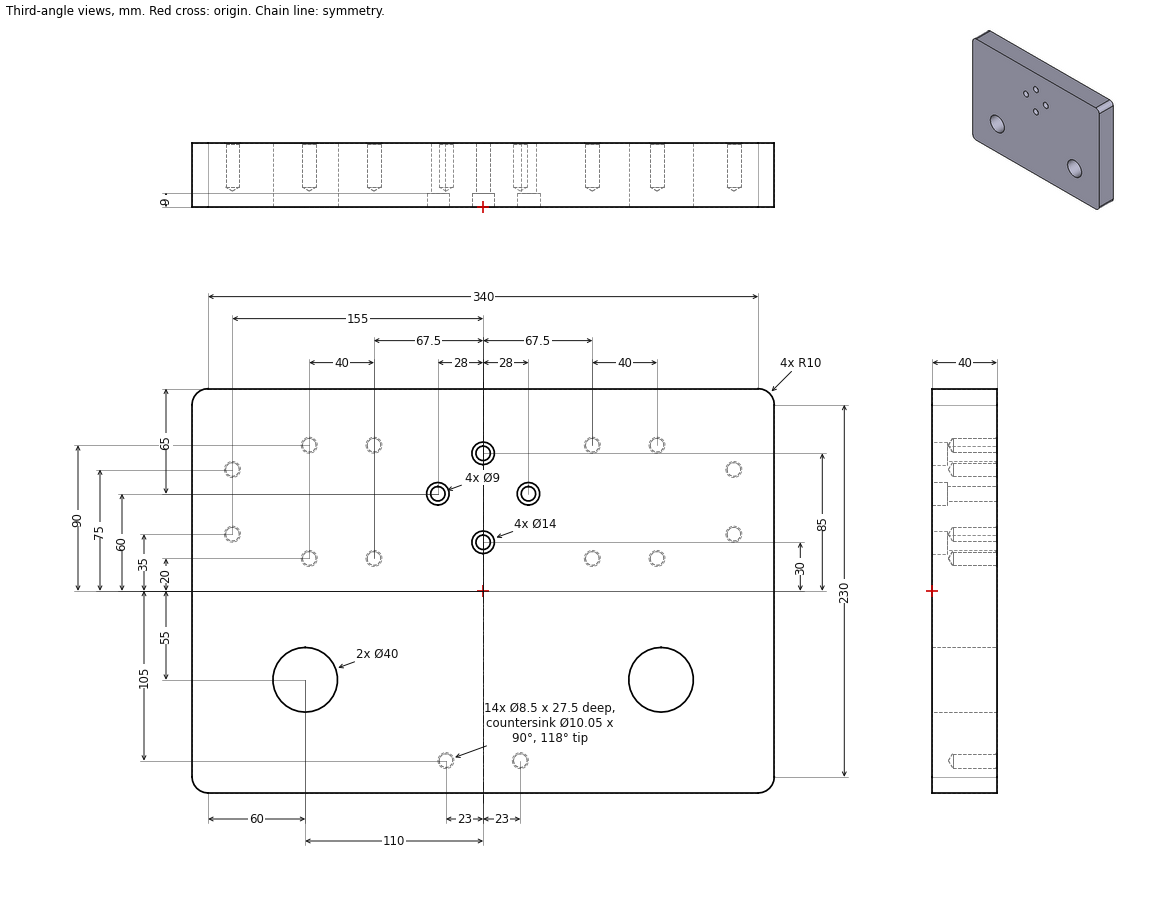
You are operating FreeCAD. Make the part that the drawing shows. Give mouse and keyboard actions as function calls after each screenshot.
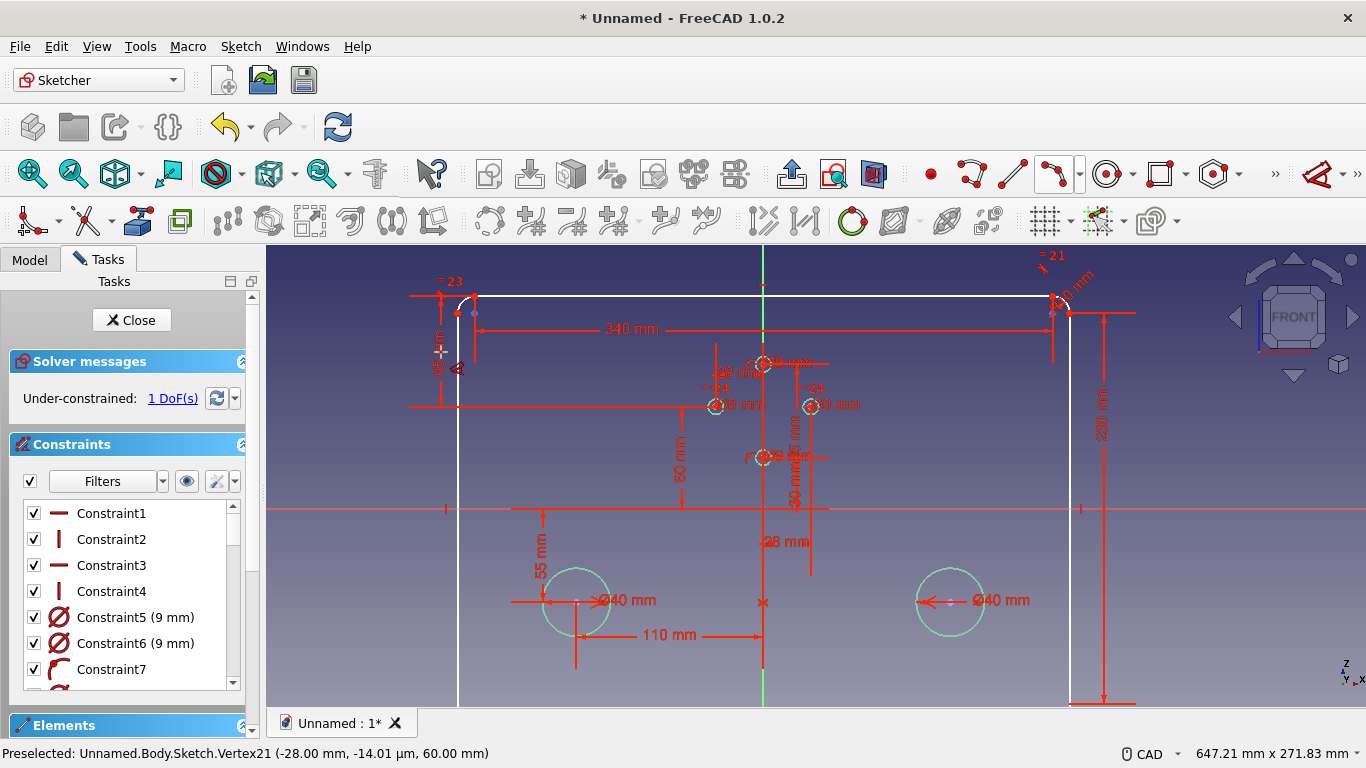
scroll(715, 409, down, 2)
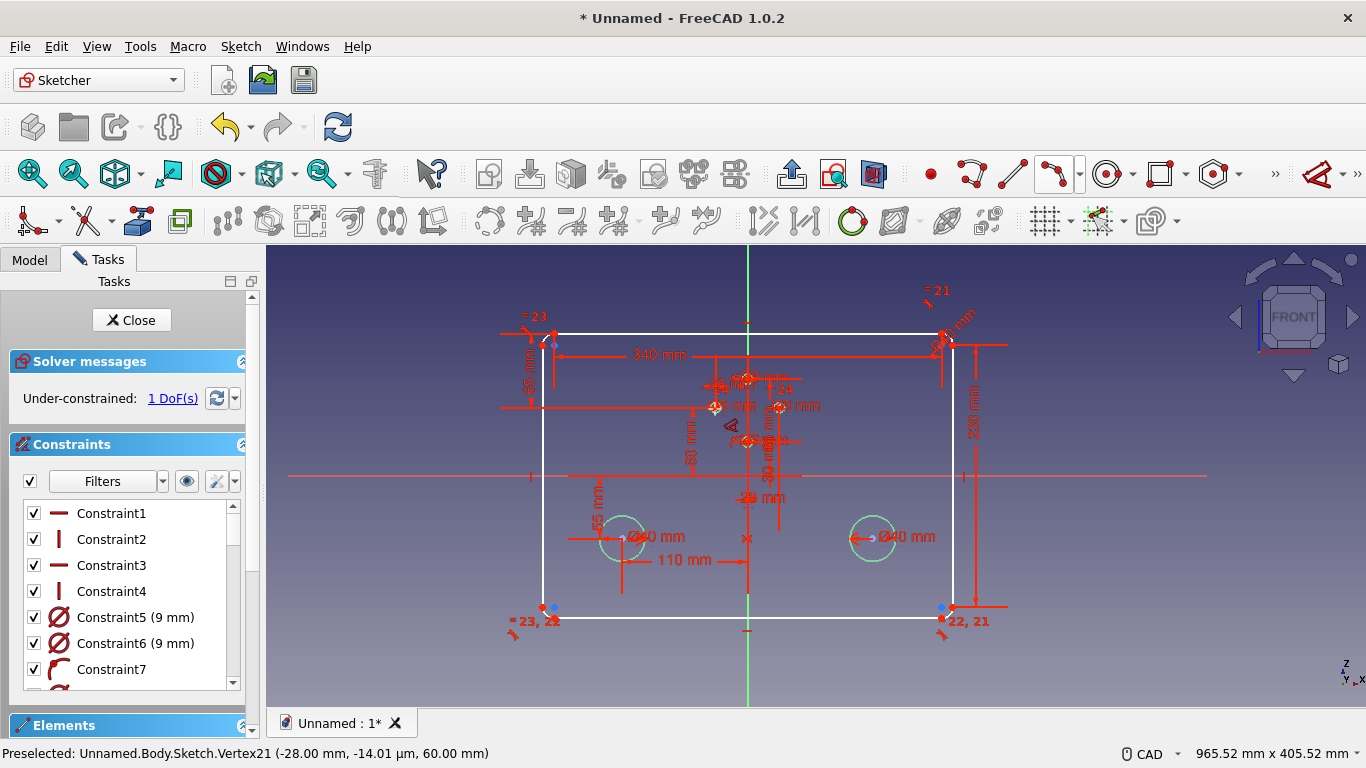
click(554, 618)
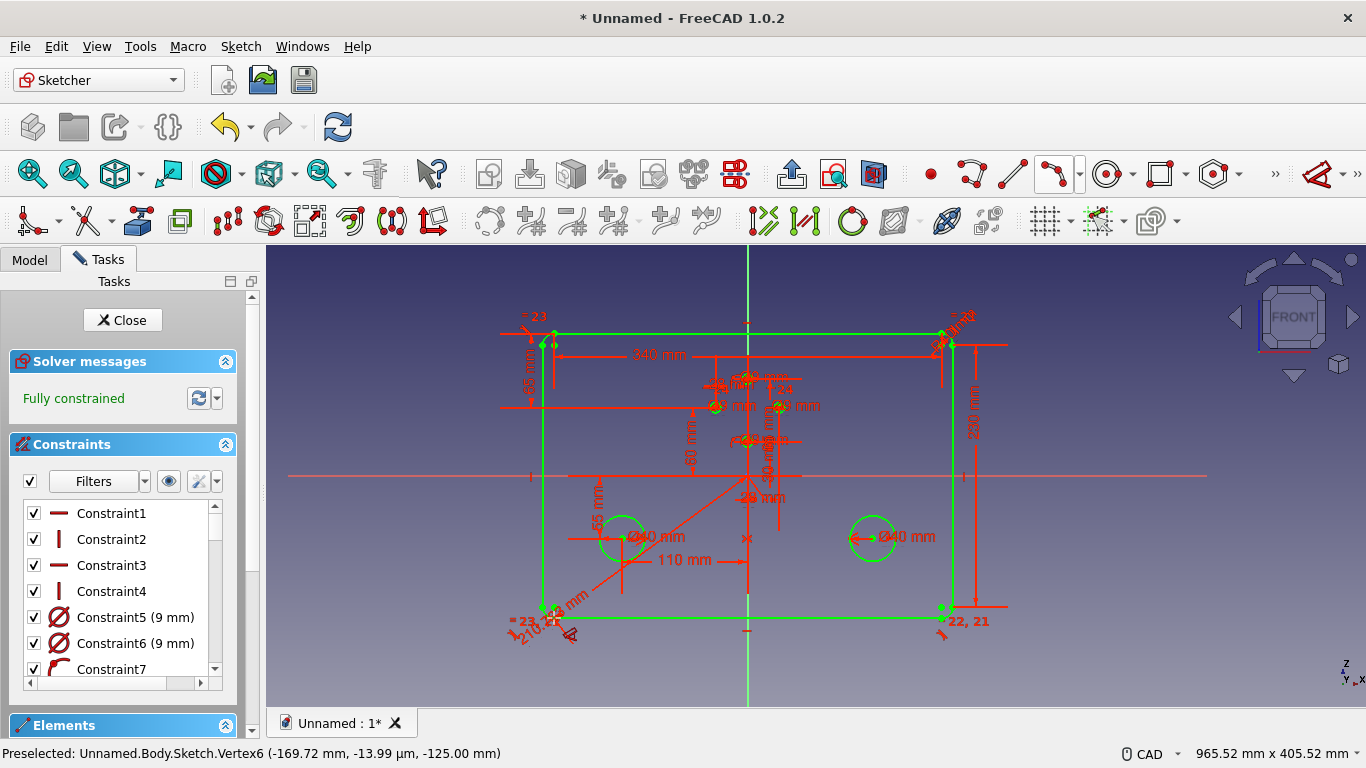
click(622, 539)
click(588, 652)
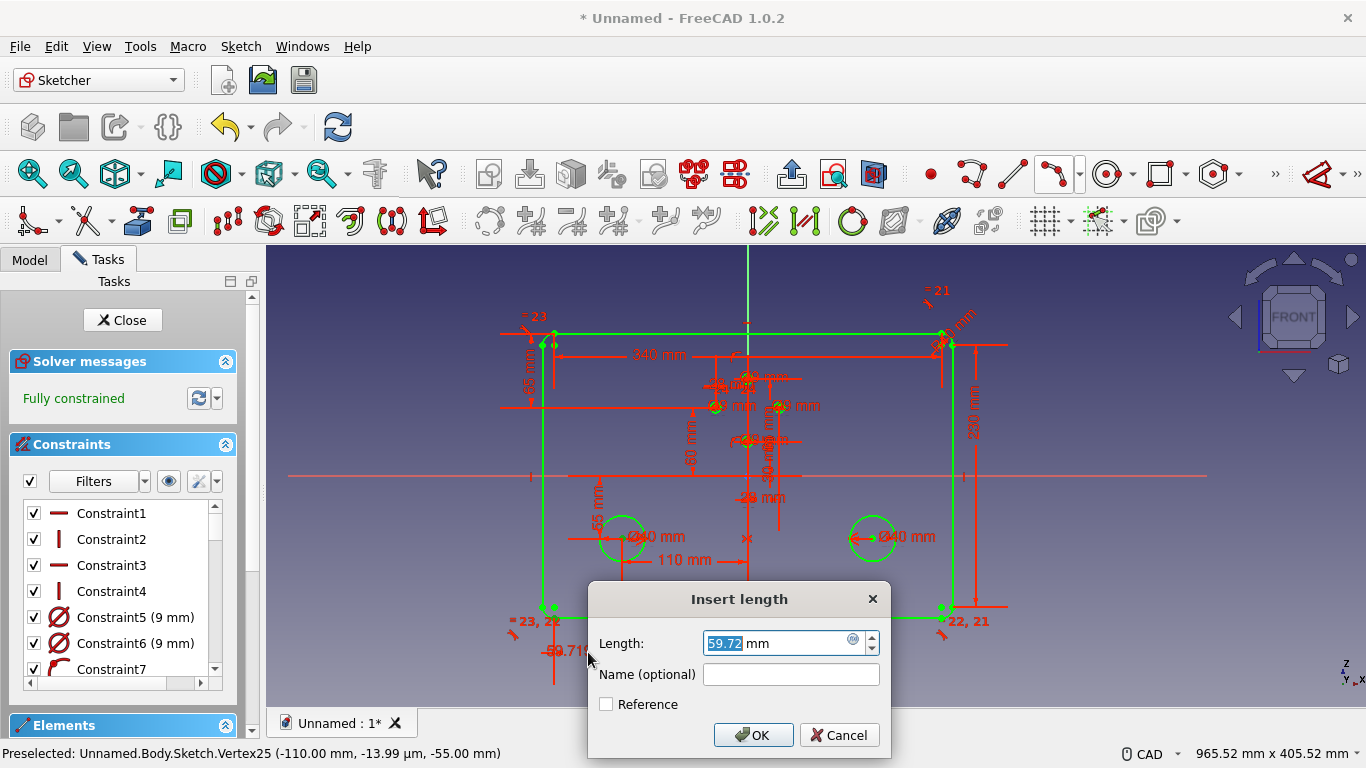
text(60)
key(Return)
key(Escape)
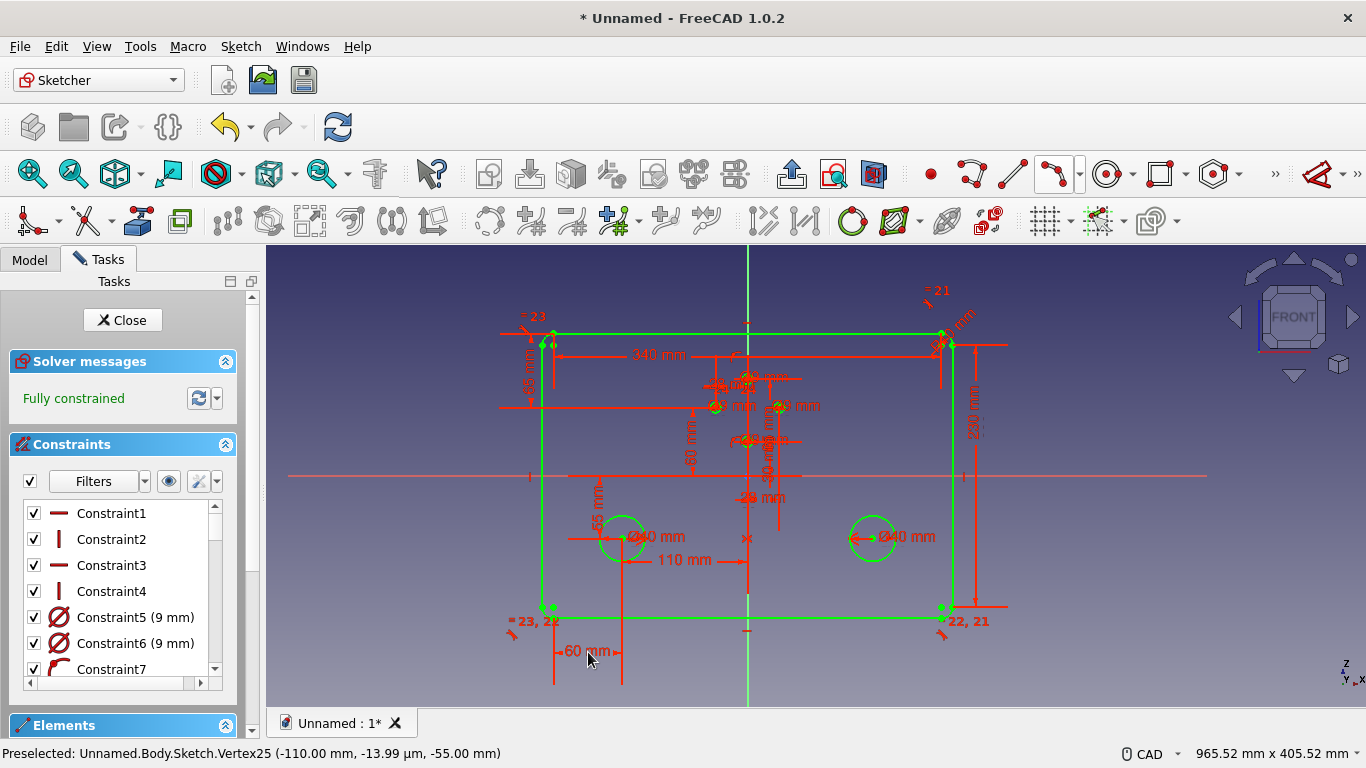
click(123, 320)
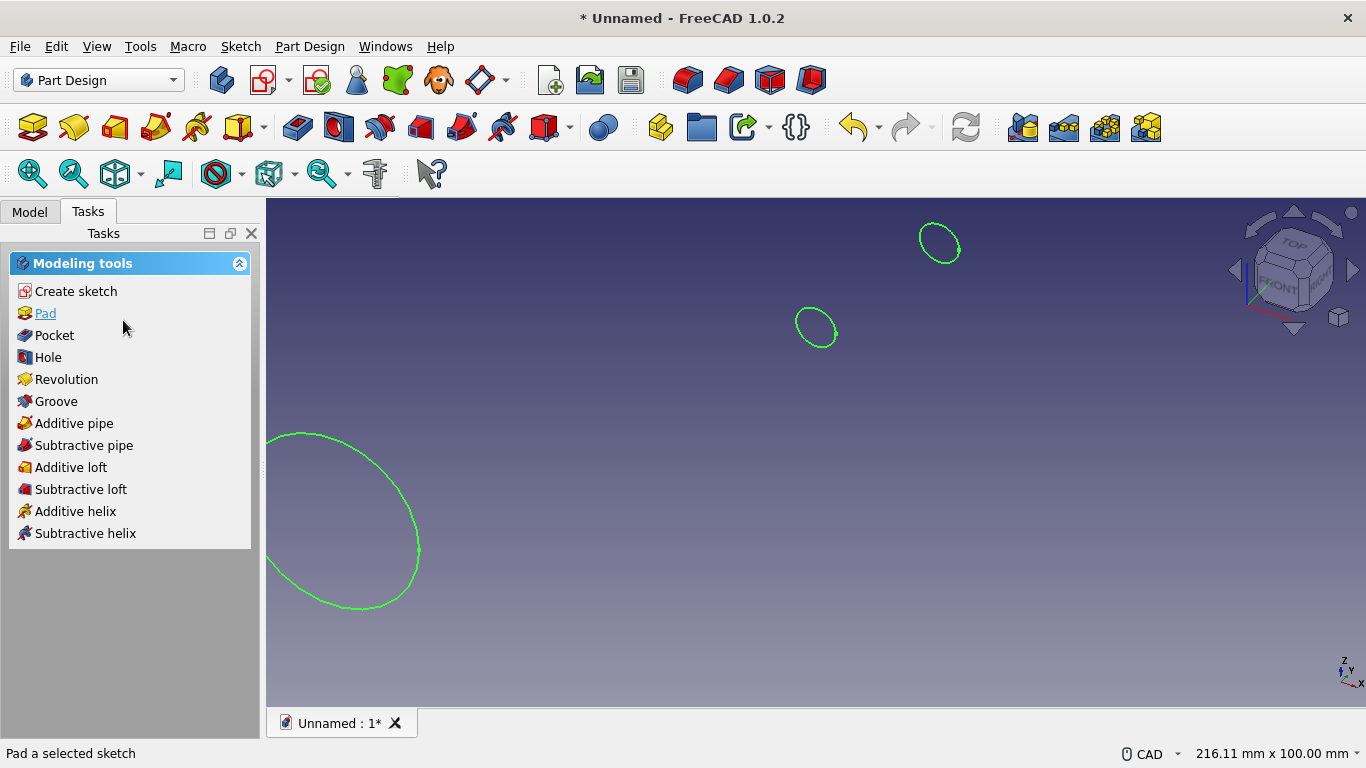
click(33, 128)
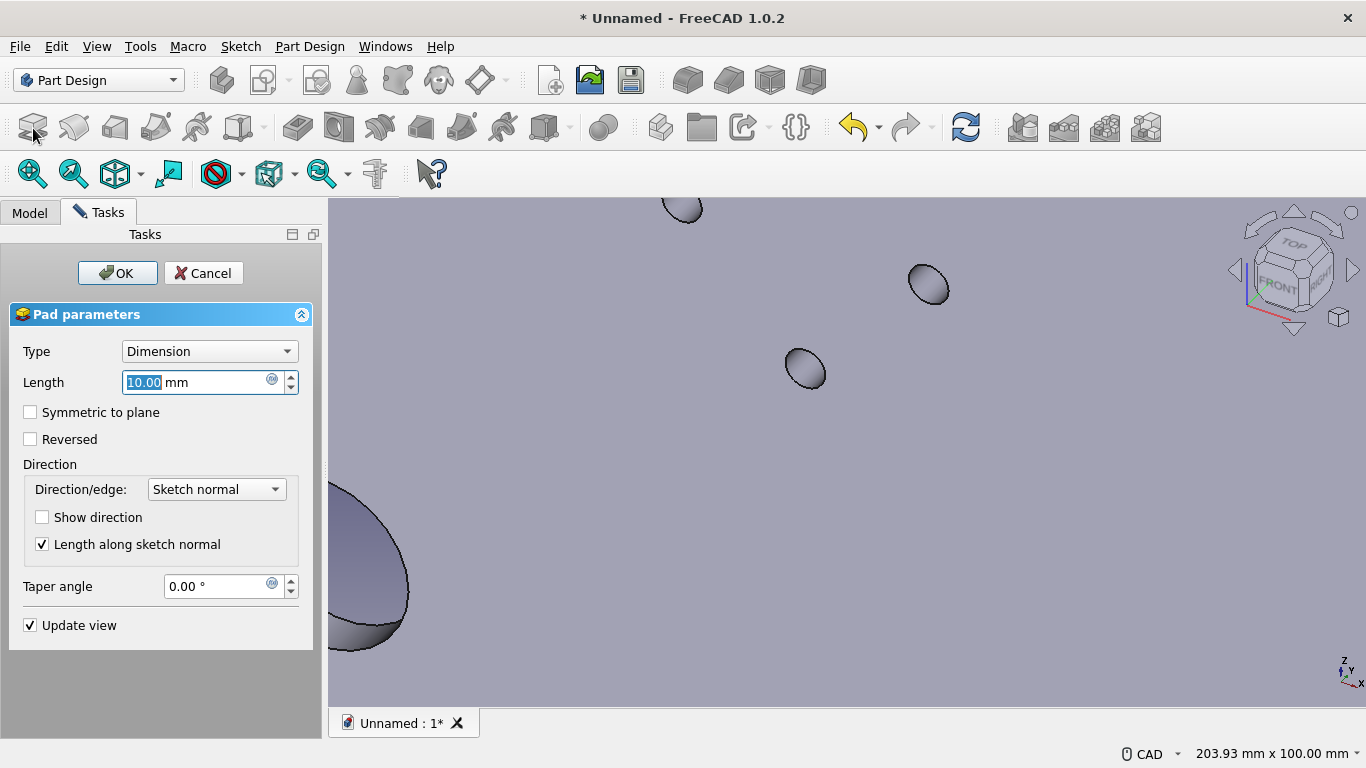
text(40)
key(Tab)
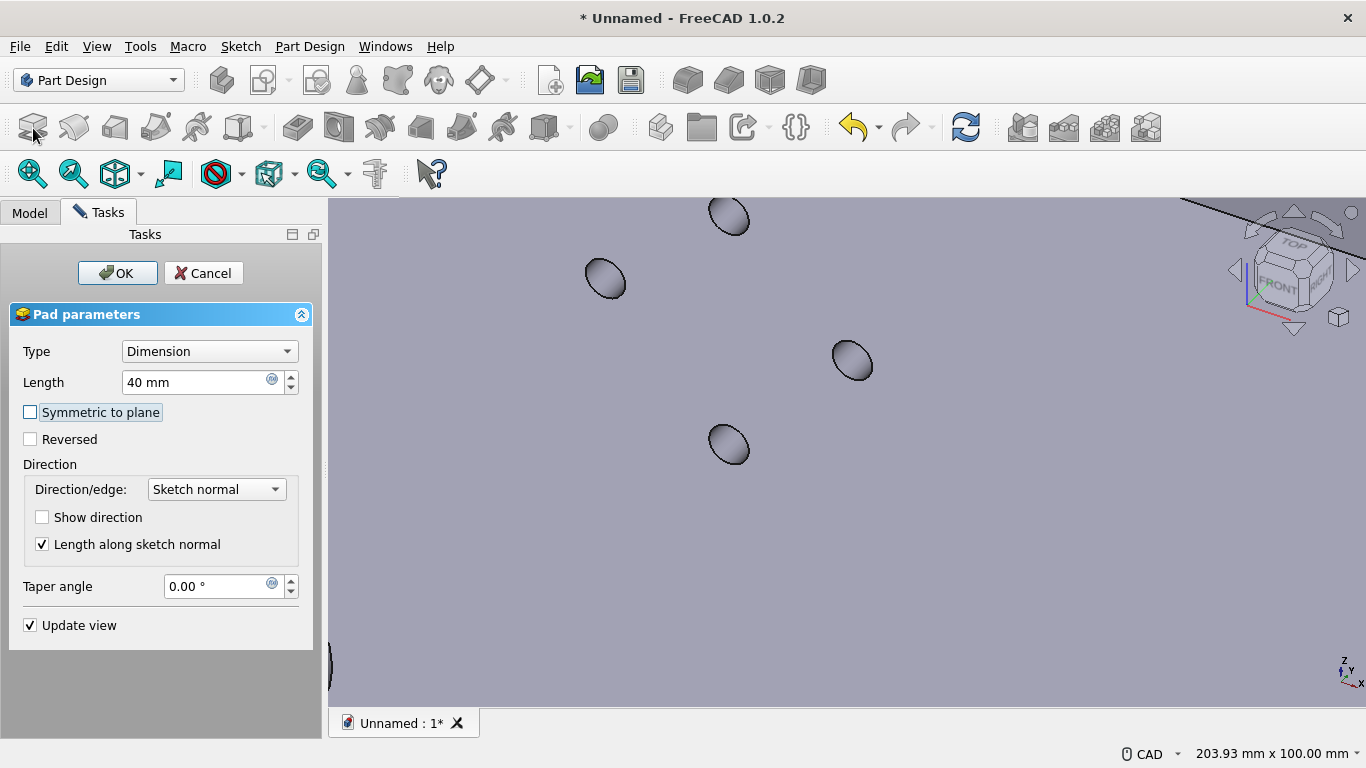
click(31, 439)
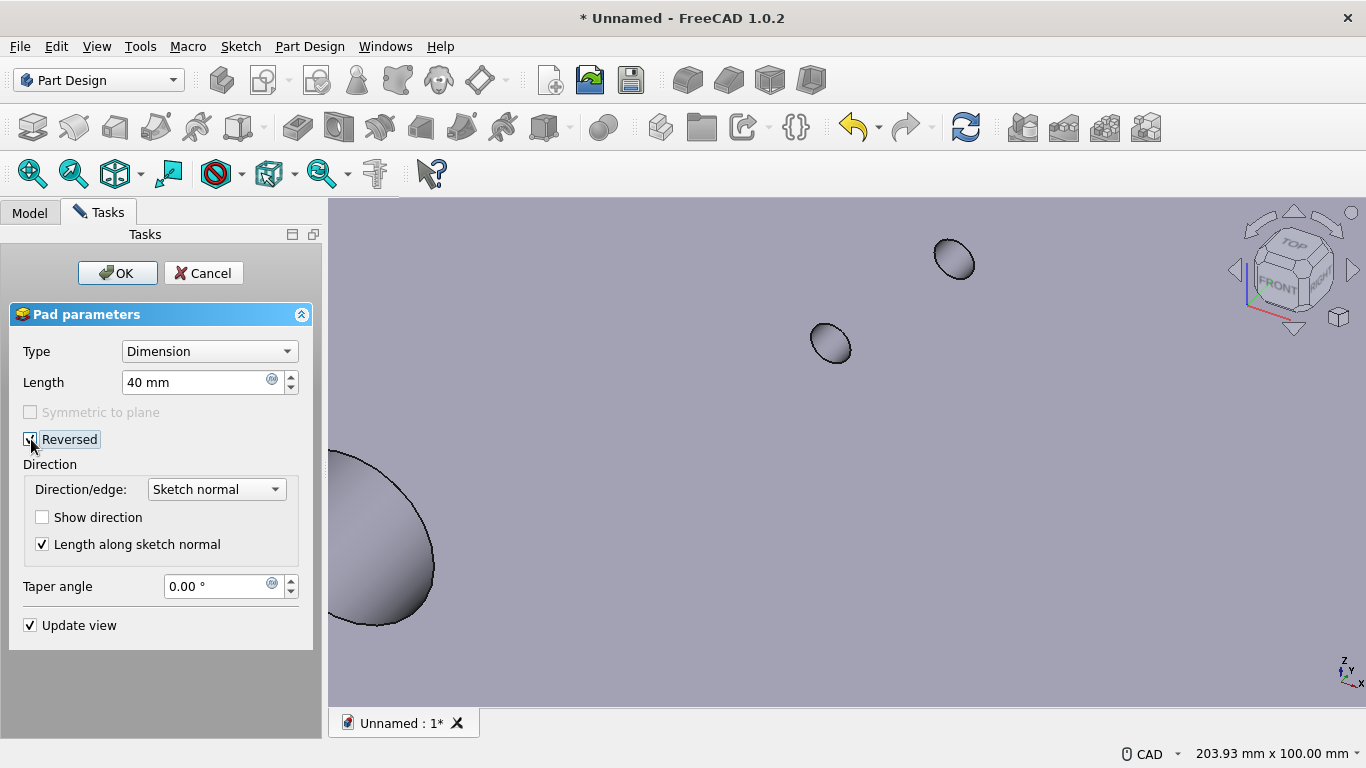
click(118, 273)